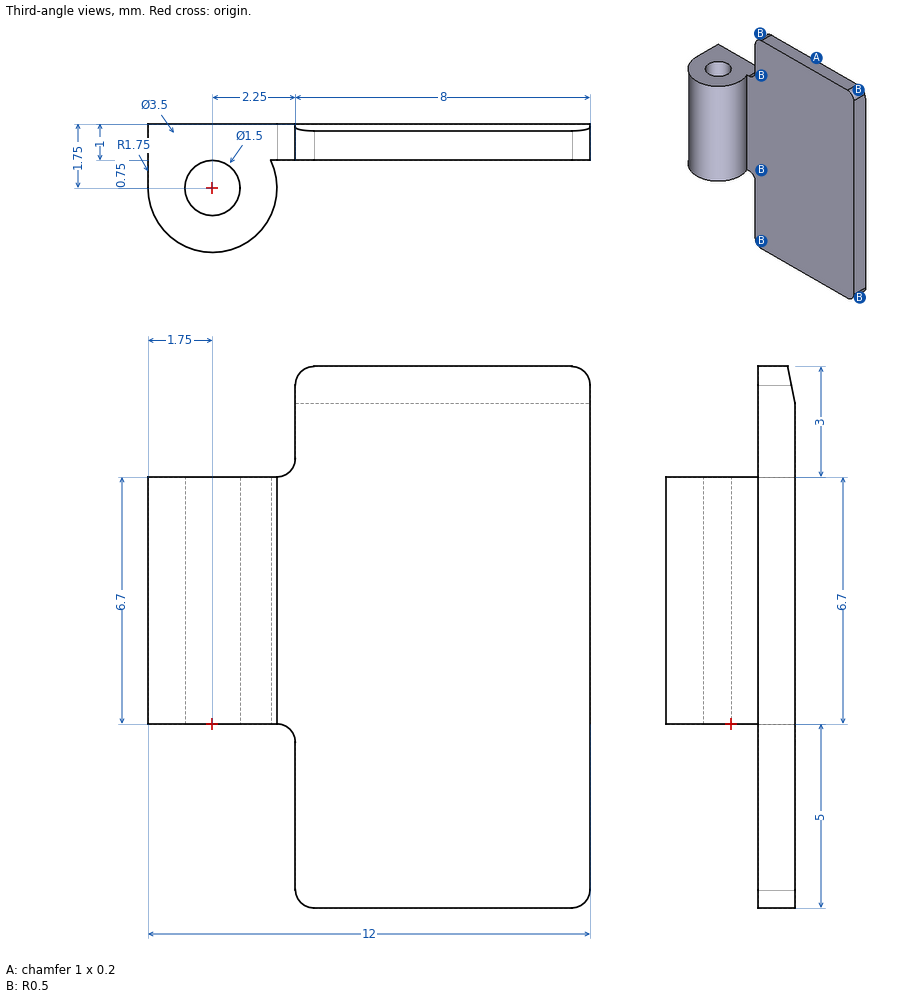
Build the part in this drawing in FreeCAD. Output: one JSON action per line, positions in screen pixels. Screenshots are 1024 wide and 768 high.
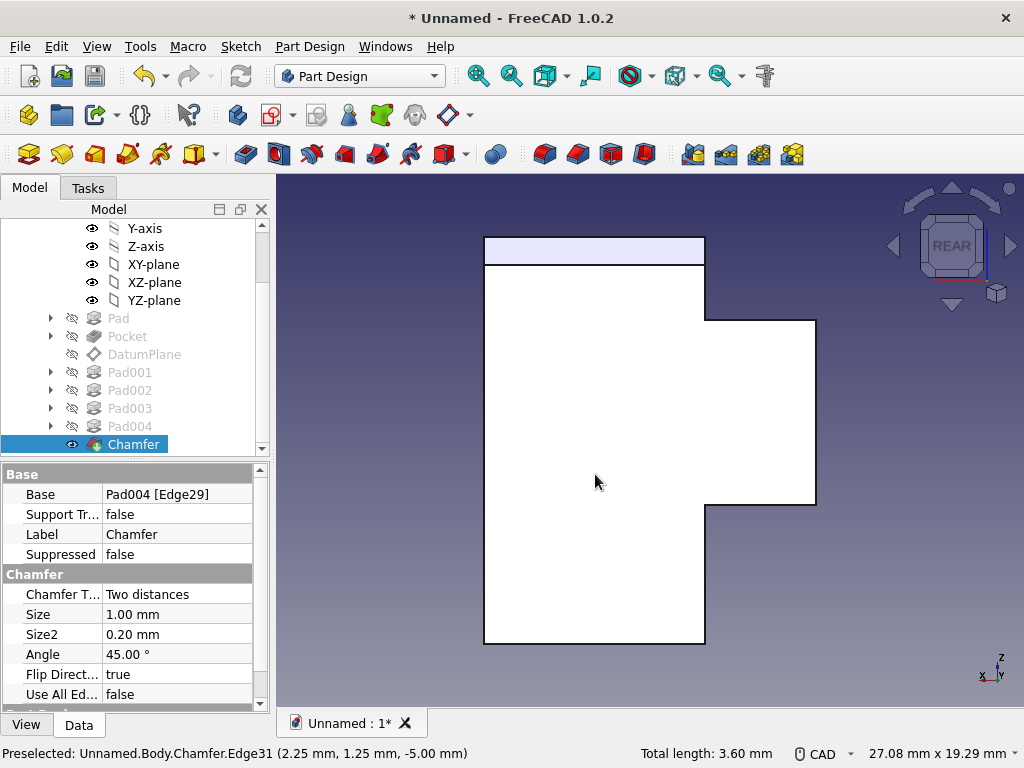
{"action": "key", "text": "6"}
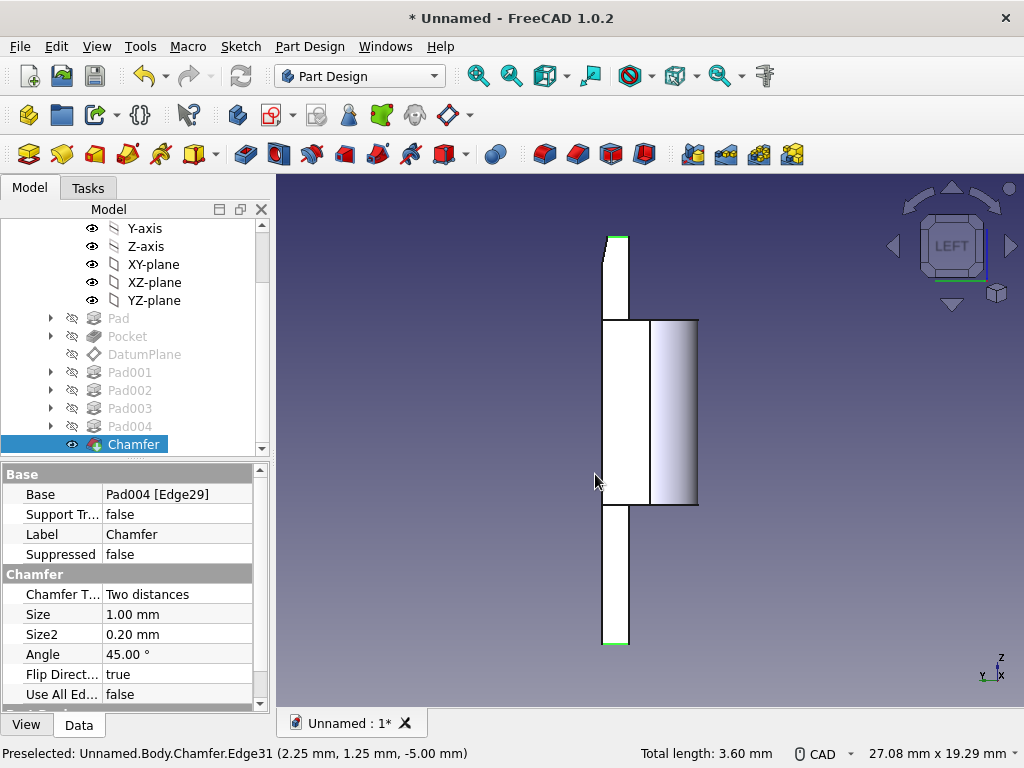
{"action": "key", "text": "v 3"}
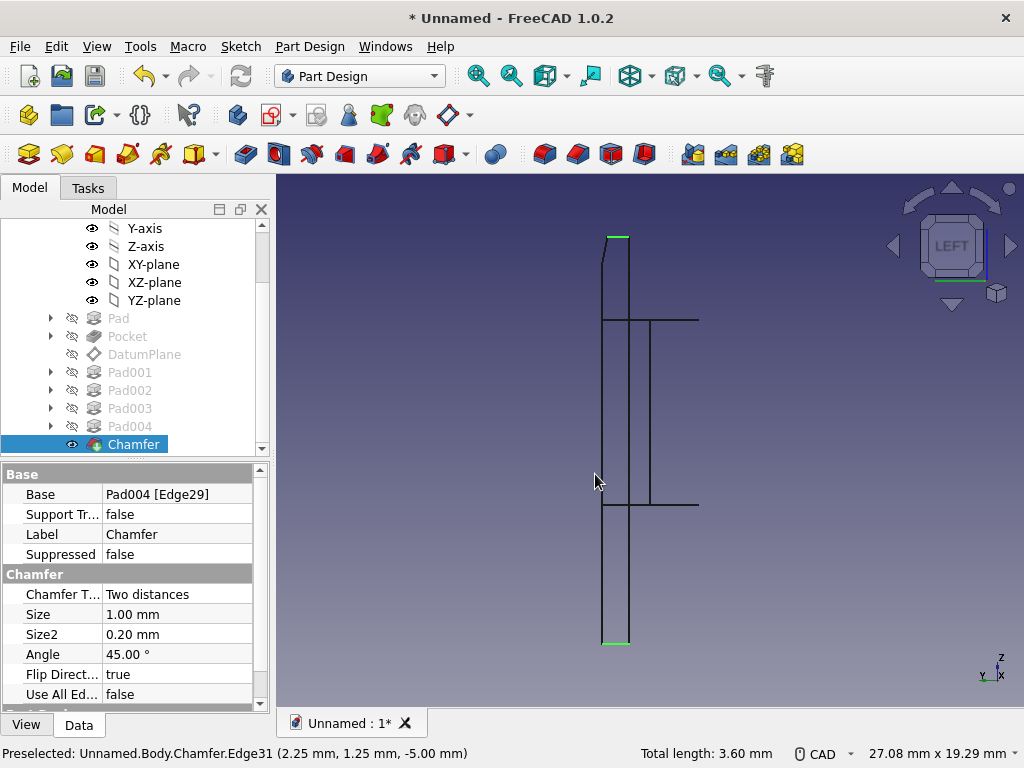
{"action": "key", "text": "0"}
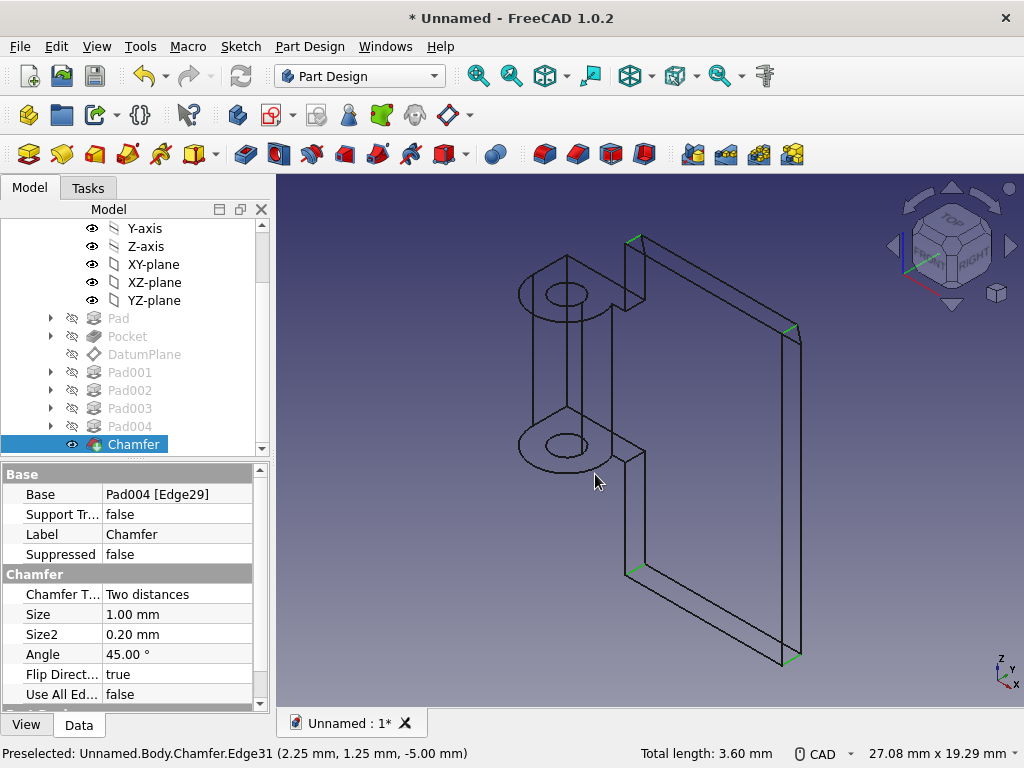
{"action": "left_click", "coordinate": [635, 305], "text": "ctrl"}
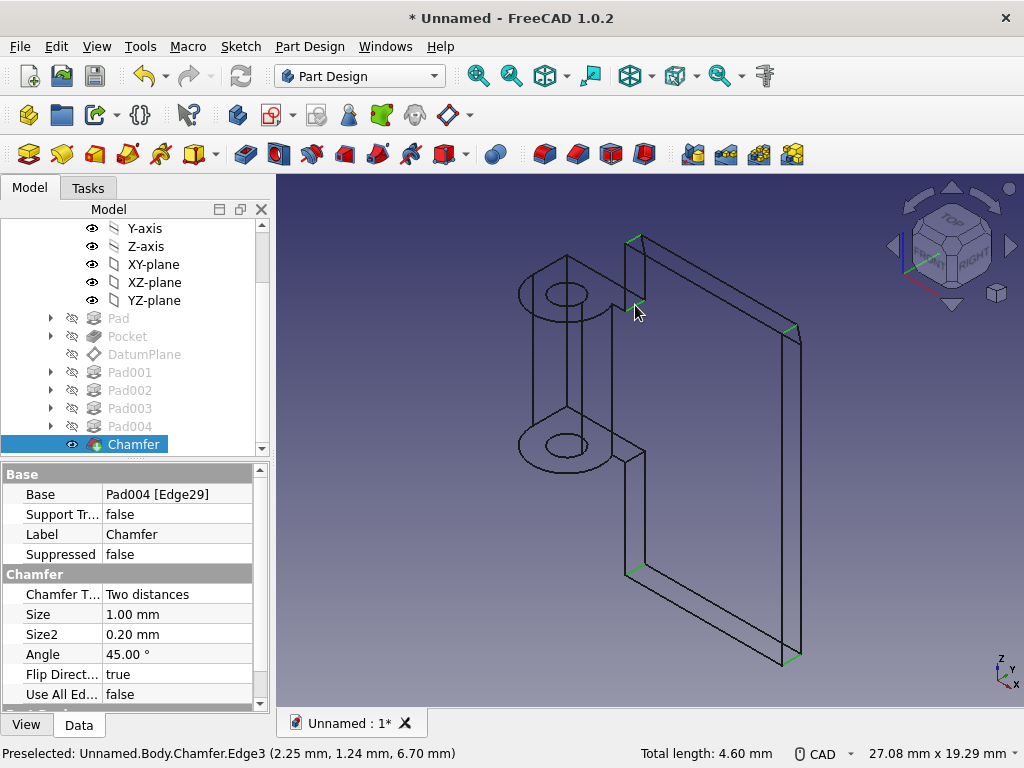
{"action": "left_click", "coordinate": [635, 456], "text": "ctrl"}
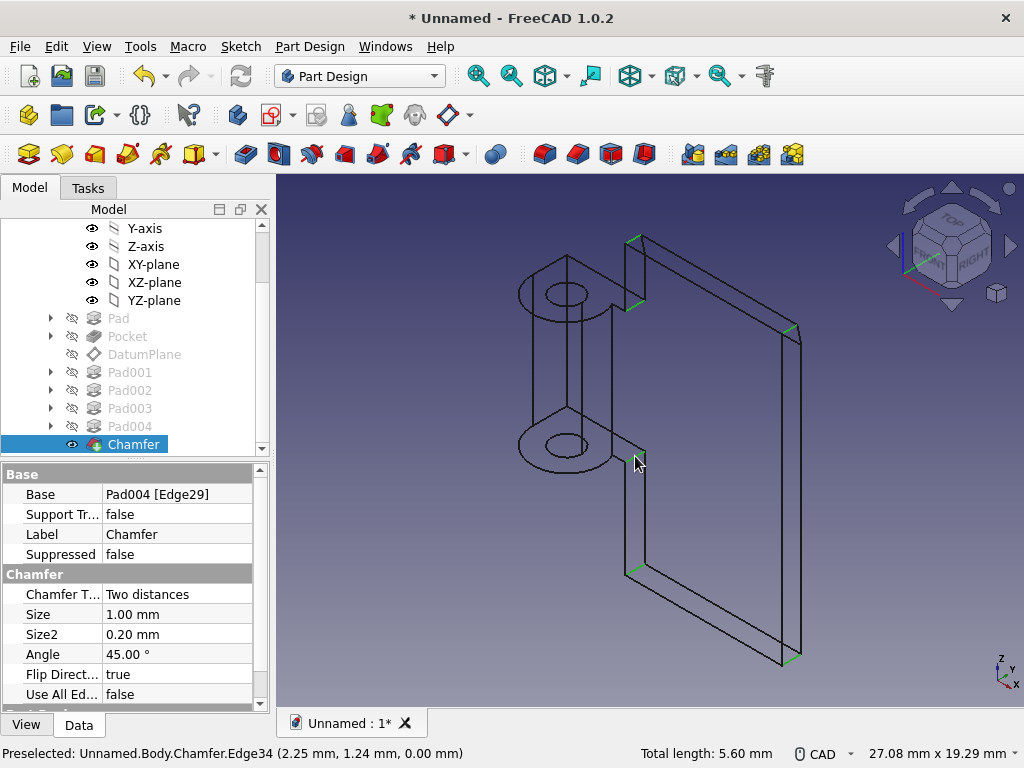
{"action": "key", "text": "v 1"}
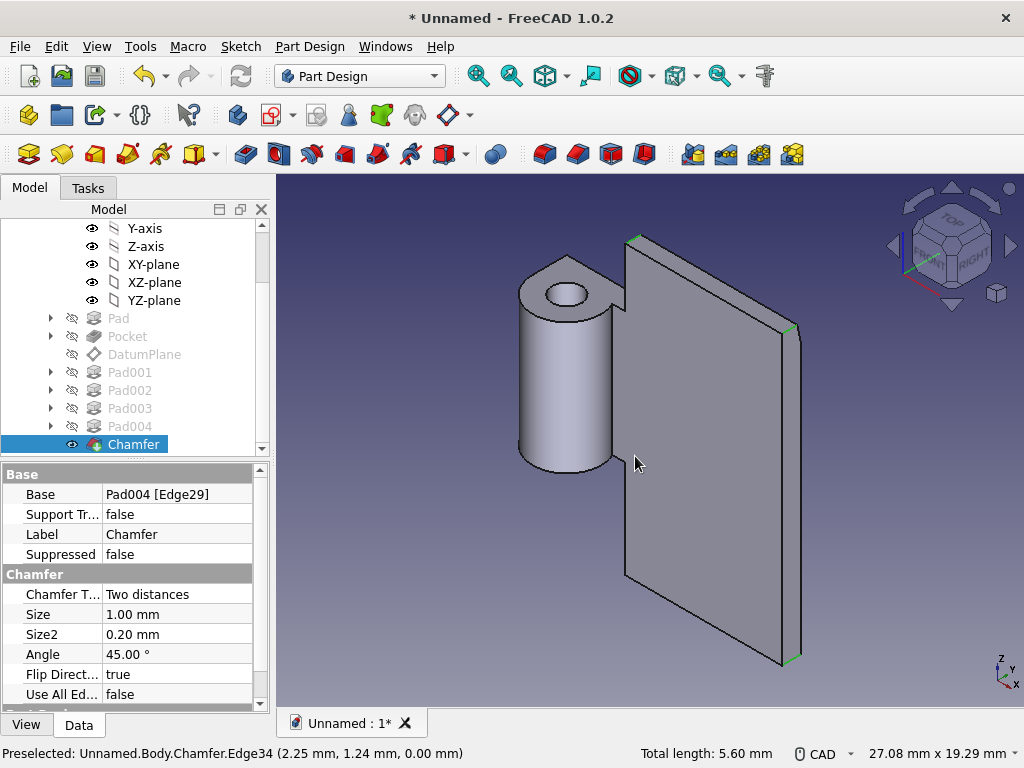
{"action": "left_click", "coordinate": [545, 154]}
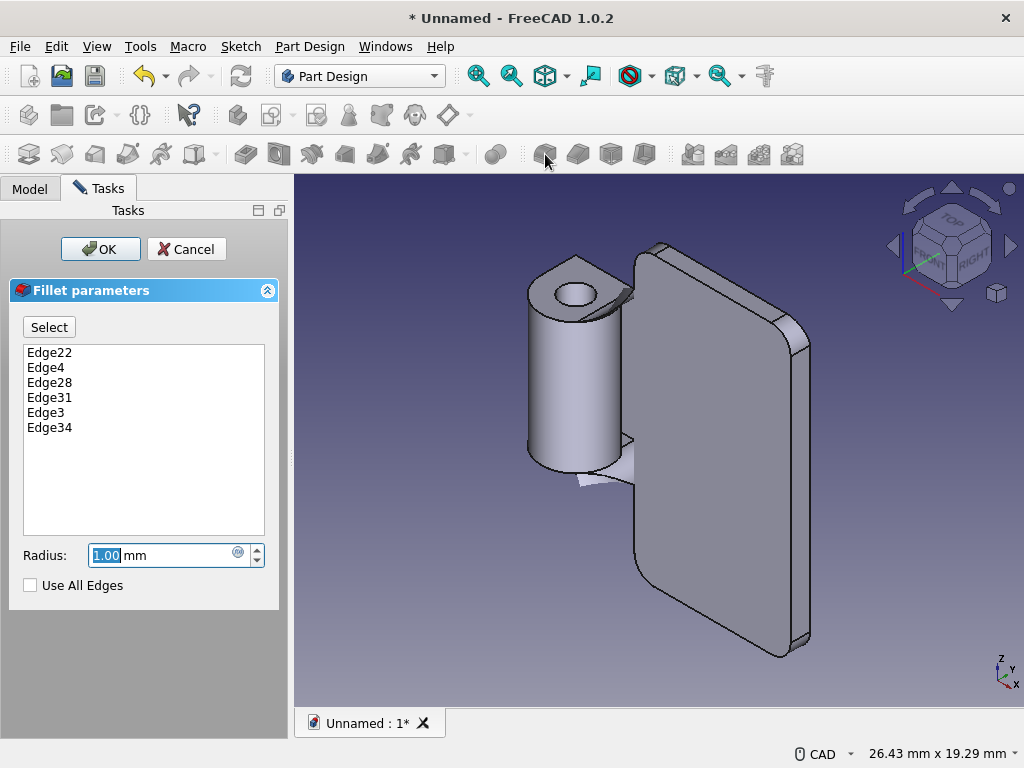
{"action": "type", "text": "0.5"}
{"action": "key", "text": "Tab"}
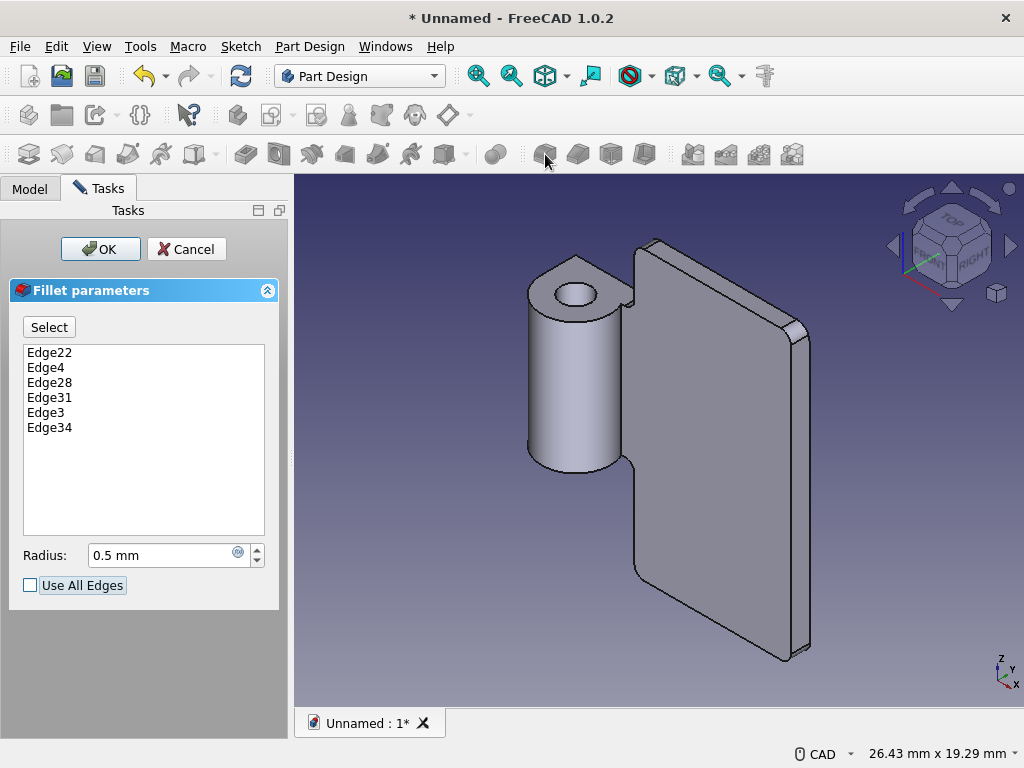
{"action": "left_click", "coordinate": [101, 249]}